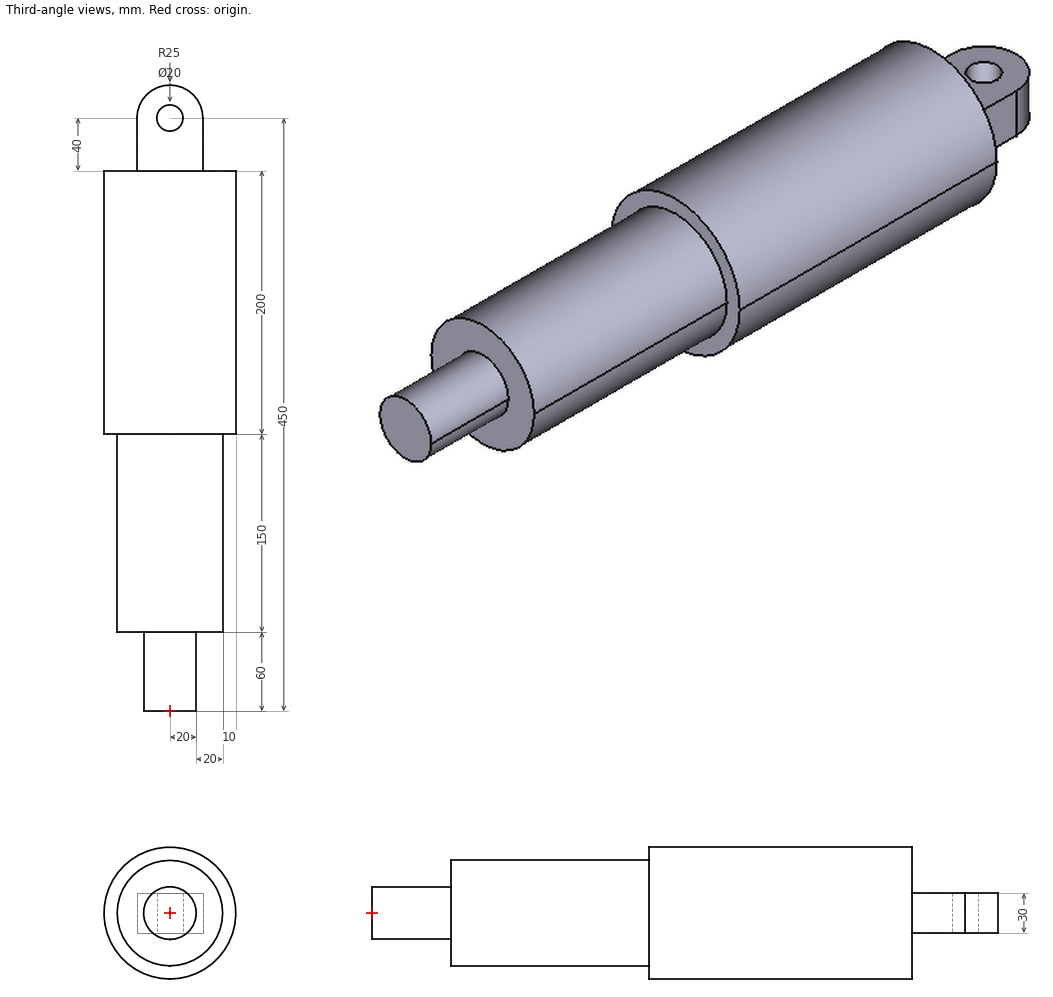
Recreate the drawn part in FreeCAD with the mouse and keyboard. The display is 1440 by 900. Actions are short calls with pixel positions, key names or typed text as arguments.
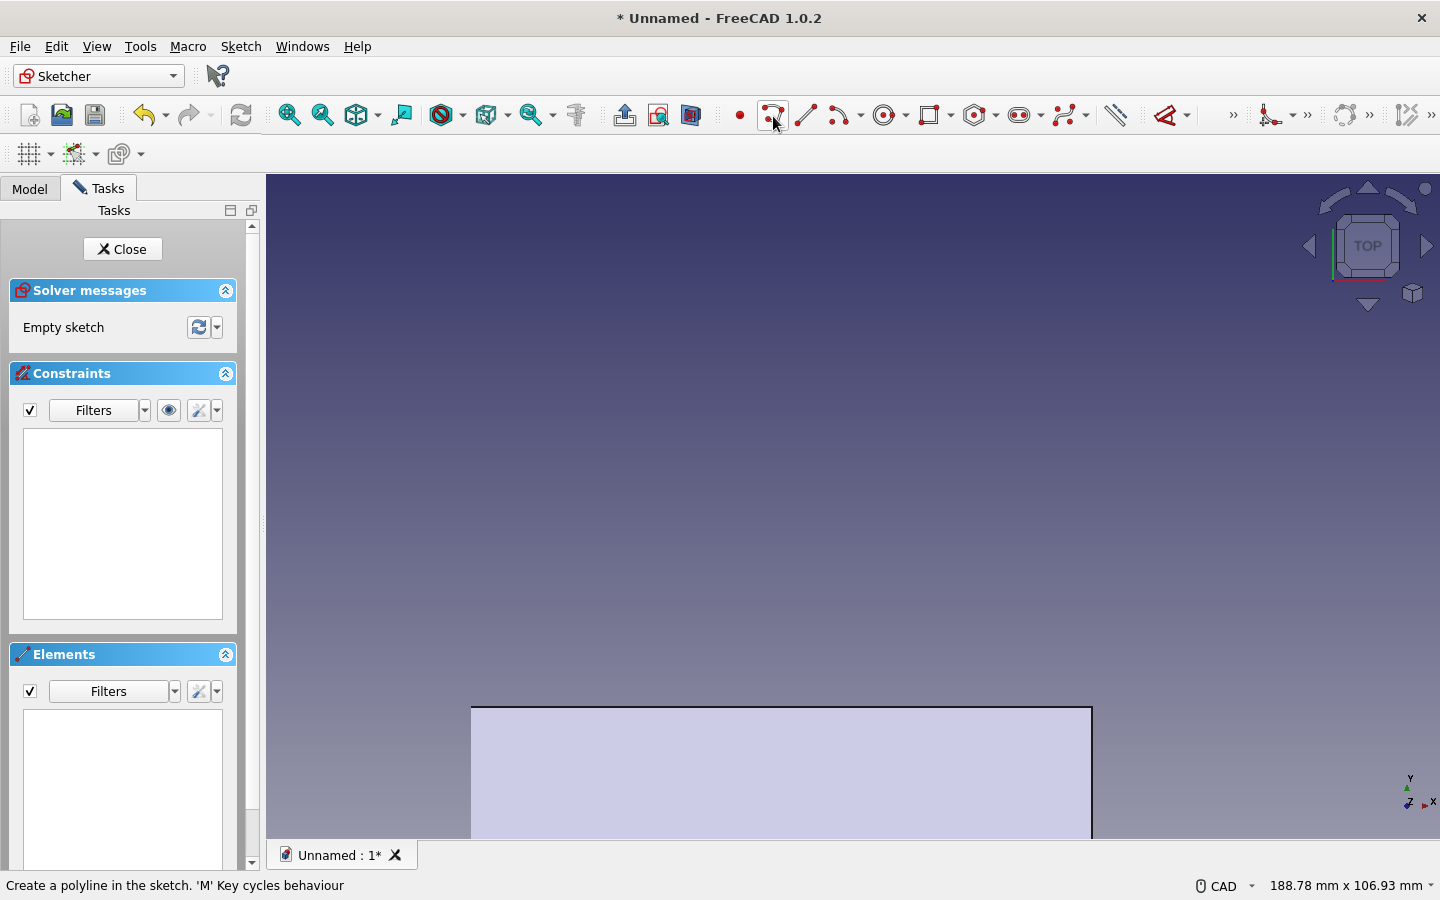
click(625, 459)
click(625, 707)
click(936, 707)
click(936, 459)
right_click(936, 459)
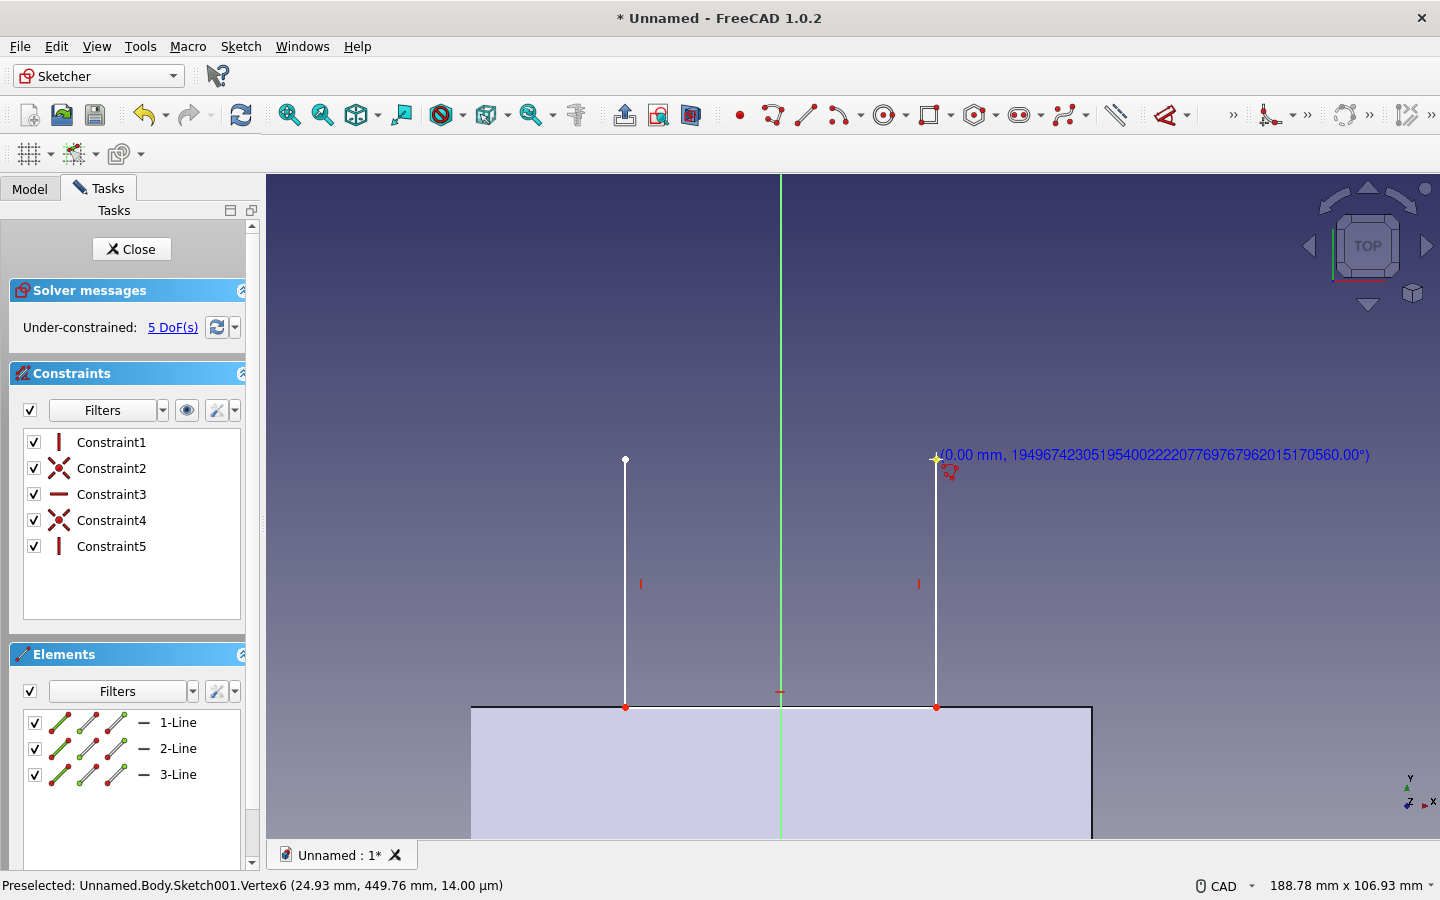
key(g)
key(3)
key(a)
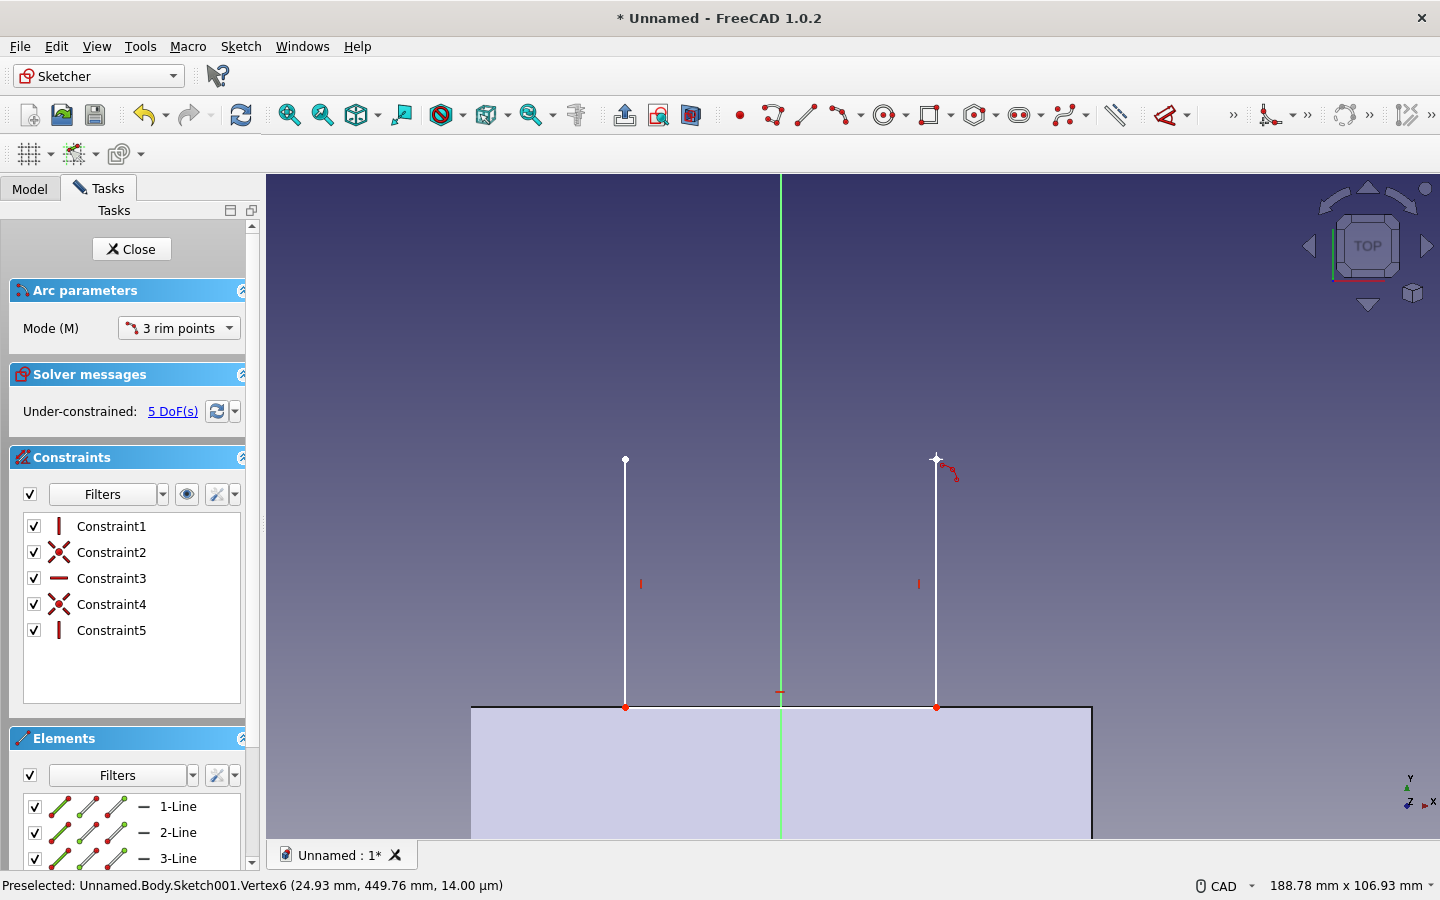
click(936, 460)
click(625, 460)
click(829, 311)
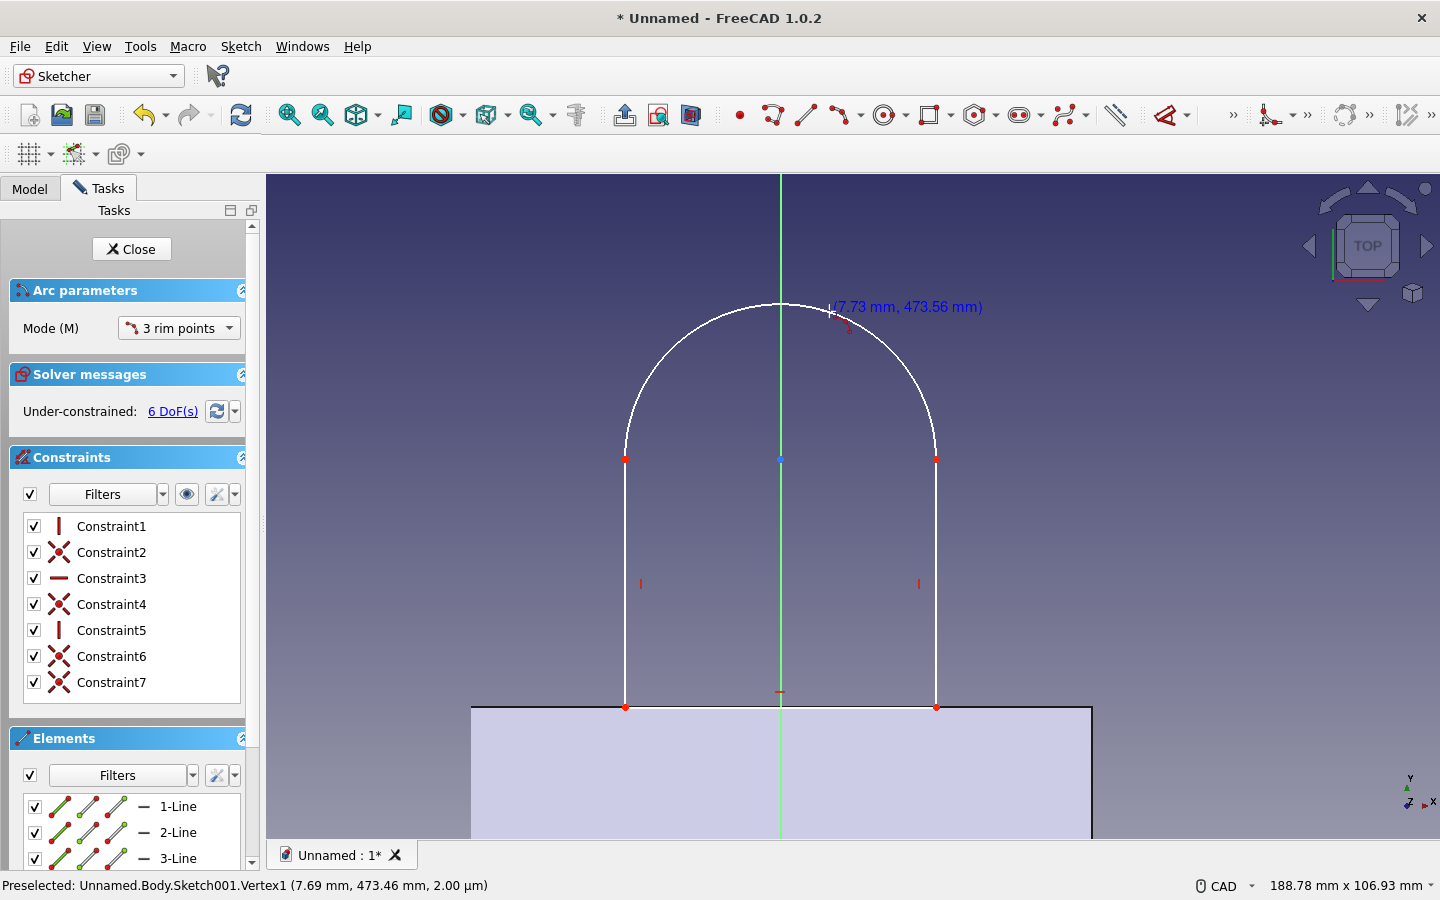
click(884, 116)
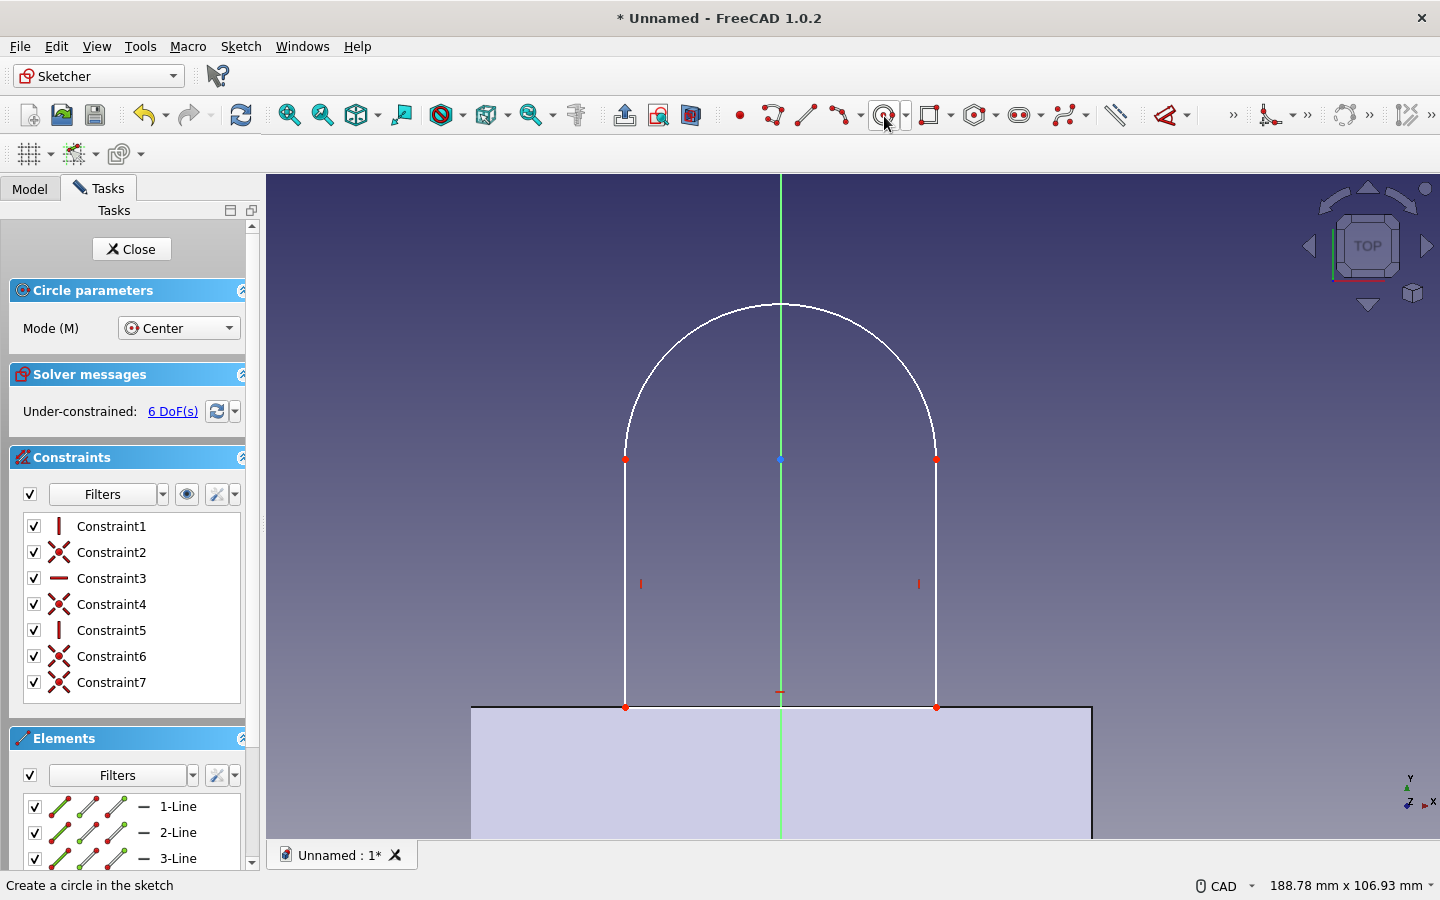
click(781, 459)
move(825, 415)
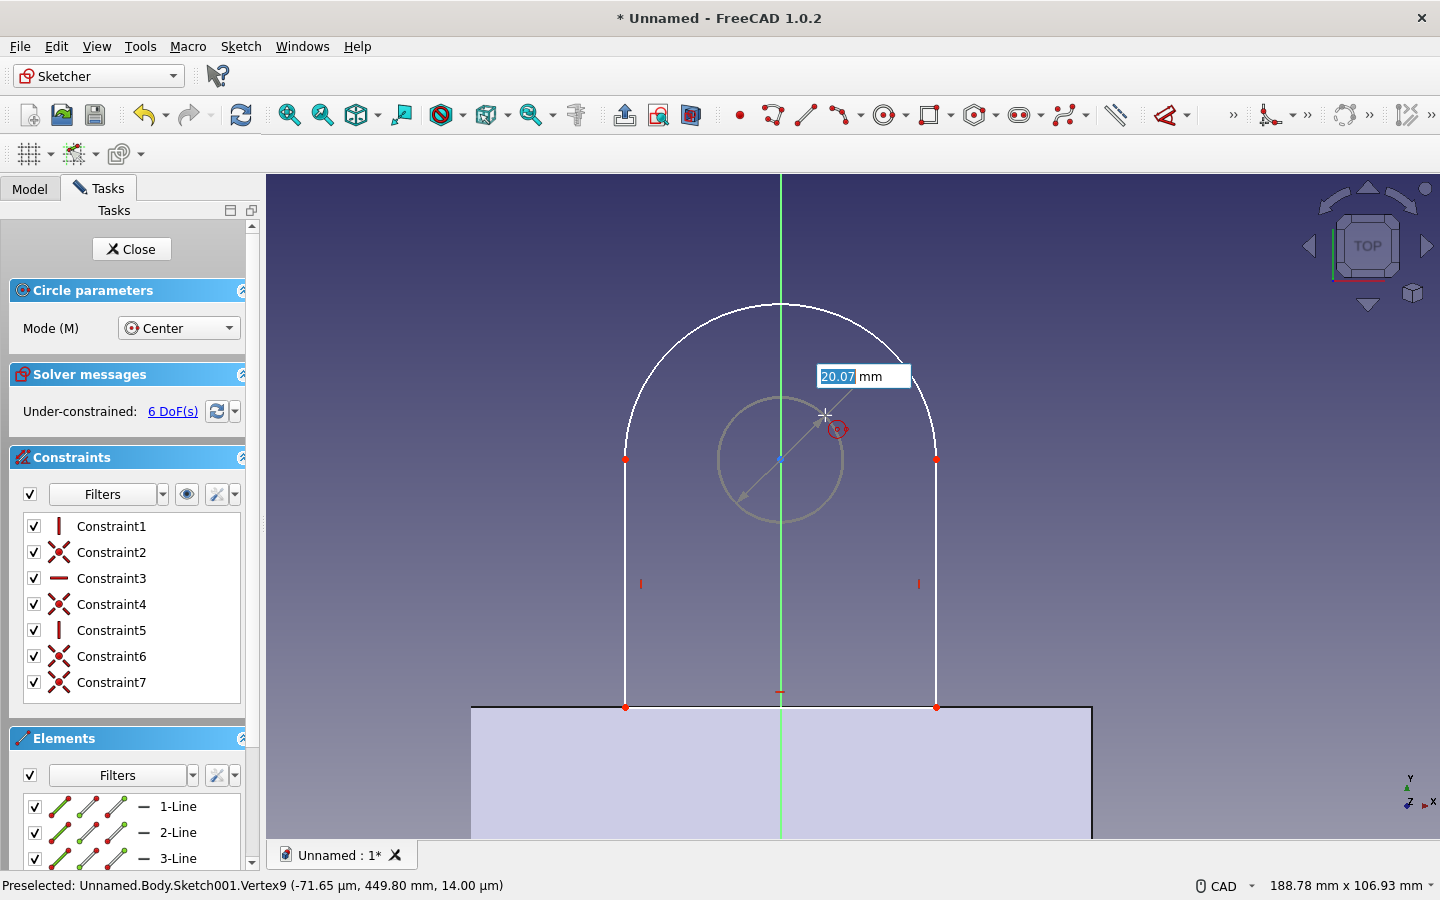
text(20)
key(Return)
key(Escape)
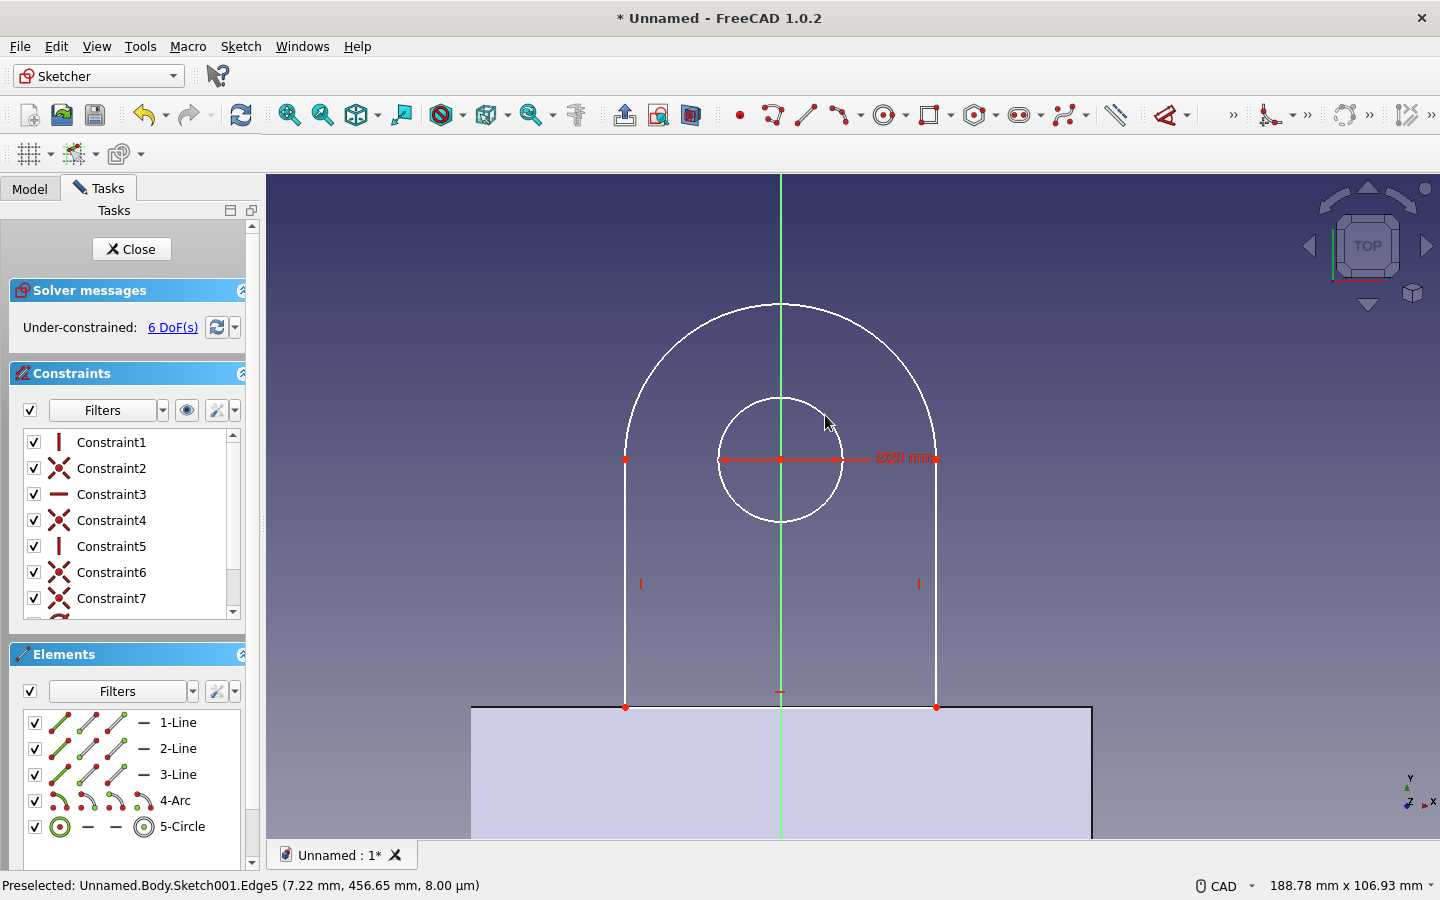
click(625, 534)